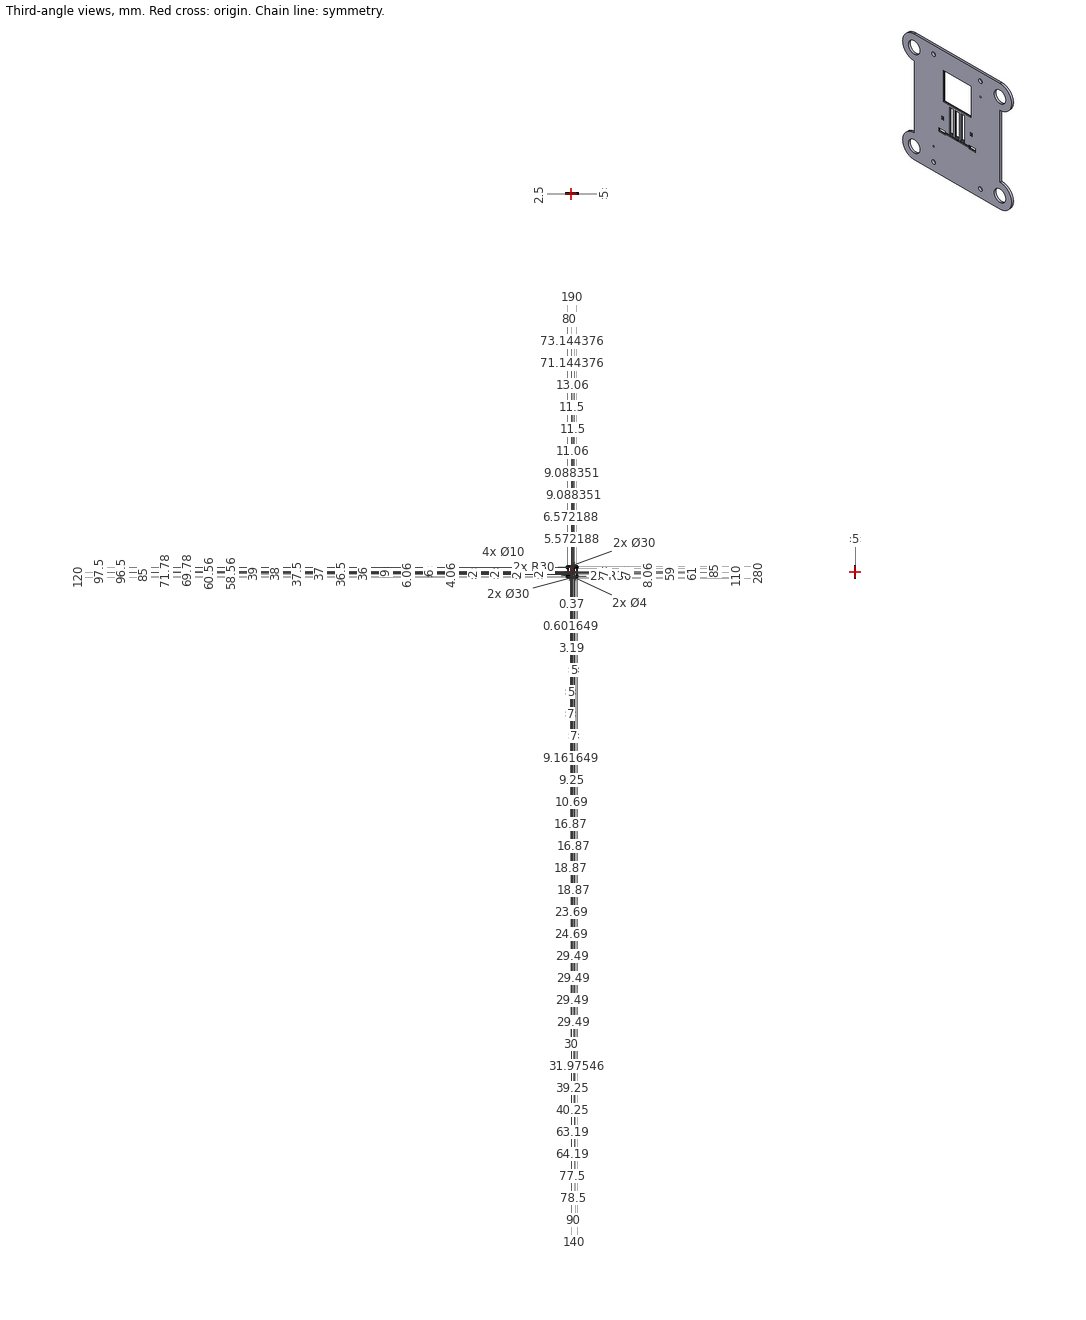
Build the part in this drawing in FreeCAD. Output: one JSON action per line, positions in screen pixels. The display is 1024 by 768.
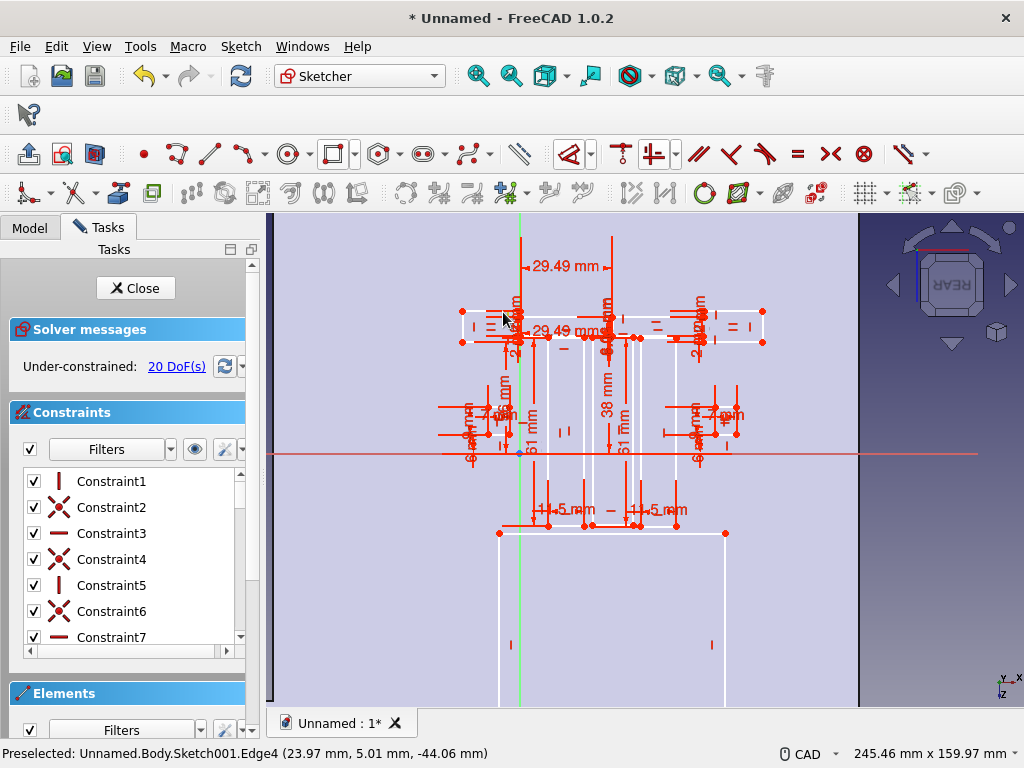
{"action": "left_click", "coordinate": [480, 311]}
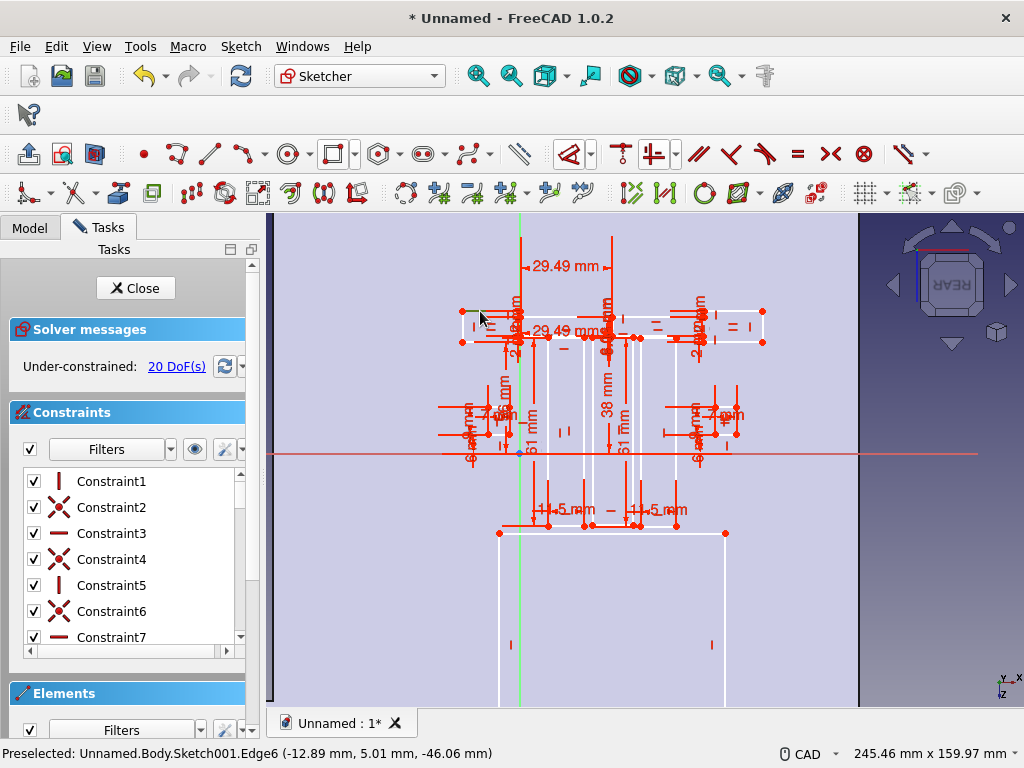
{"action": "key", "text": "l"}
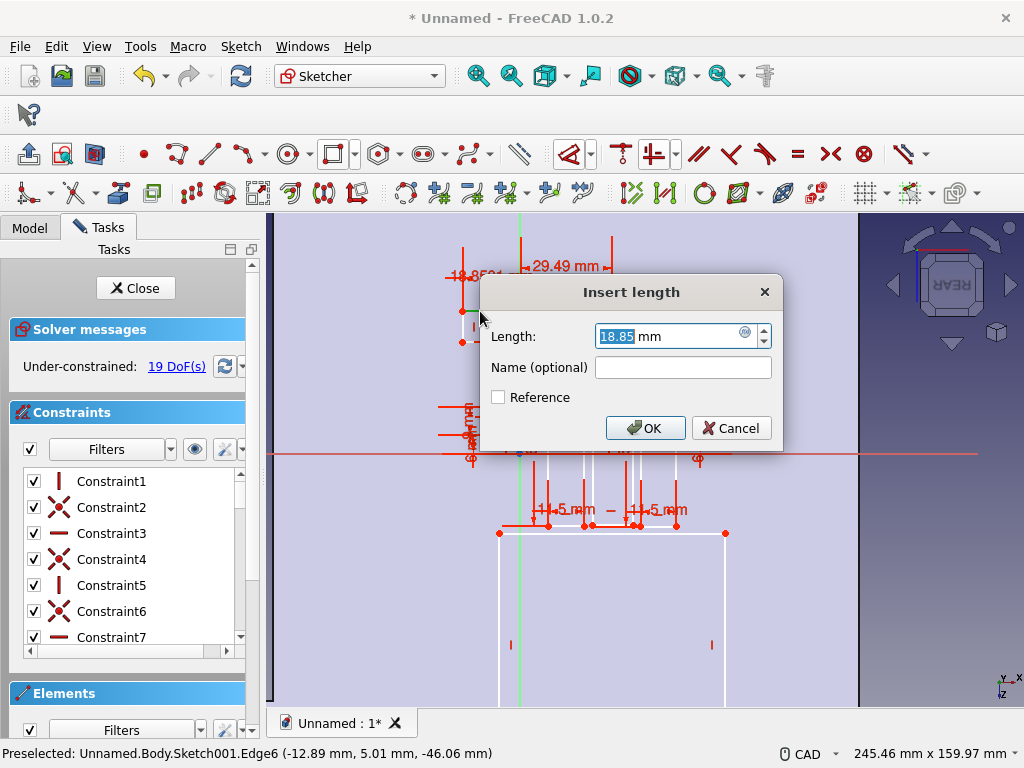
{"action": "type", "text": "18.87"}
{"action": "key", "text": "Return"}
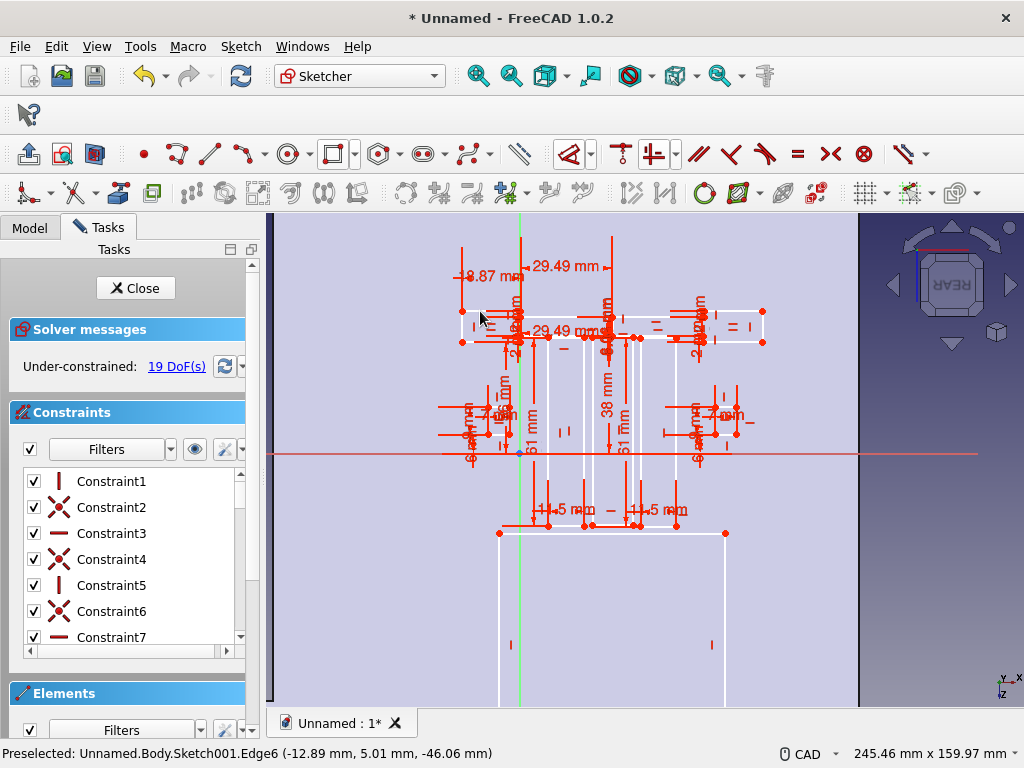
{"action": "left_click", "coordinate": [499, 600]}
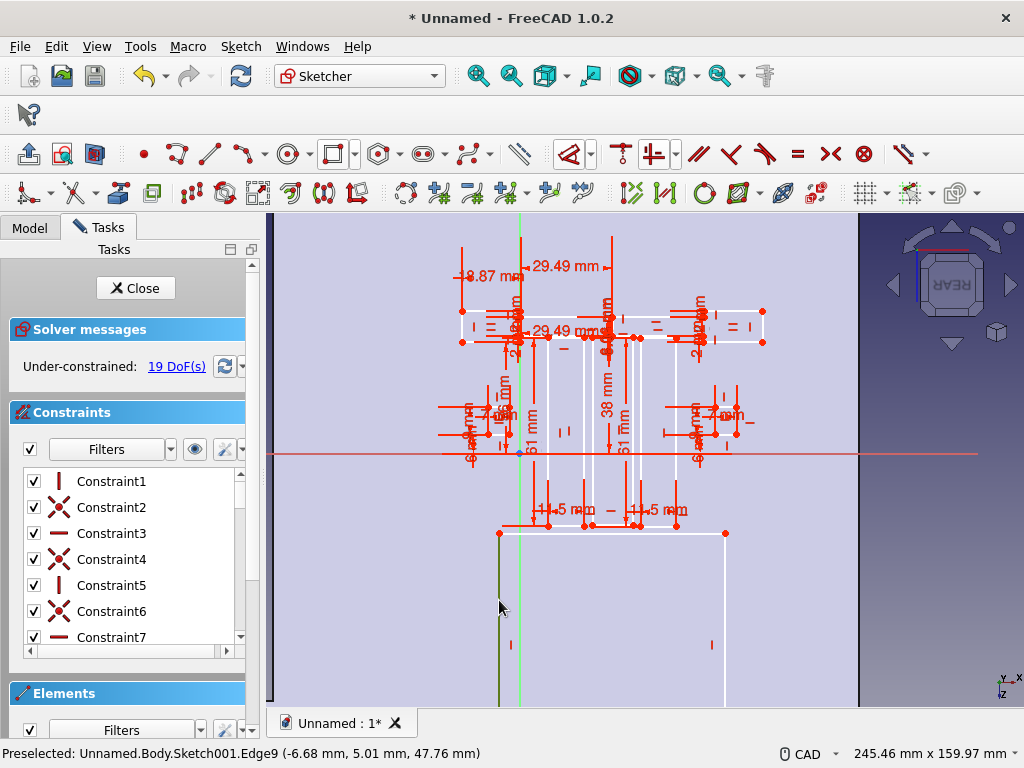
{"action": "key", "text": "i"}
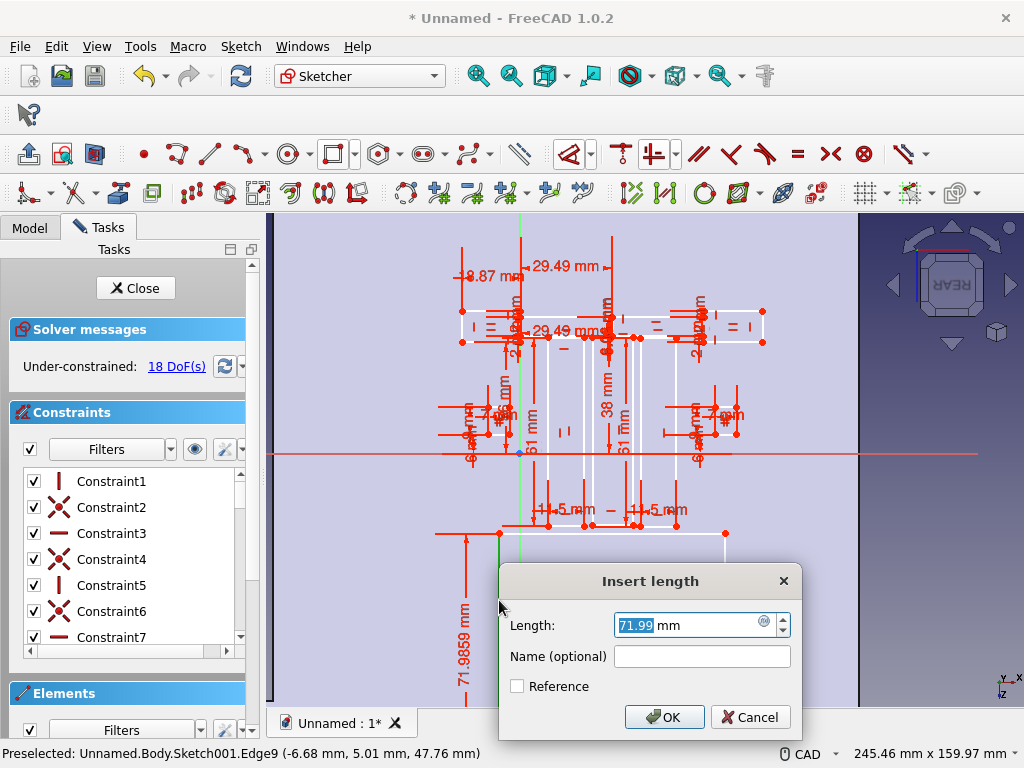
{"action": "type", "text": "71.78"}
{"action": "key", "text": "Return"}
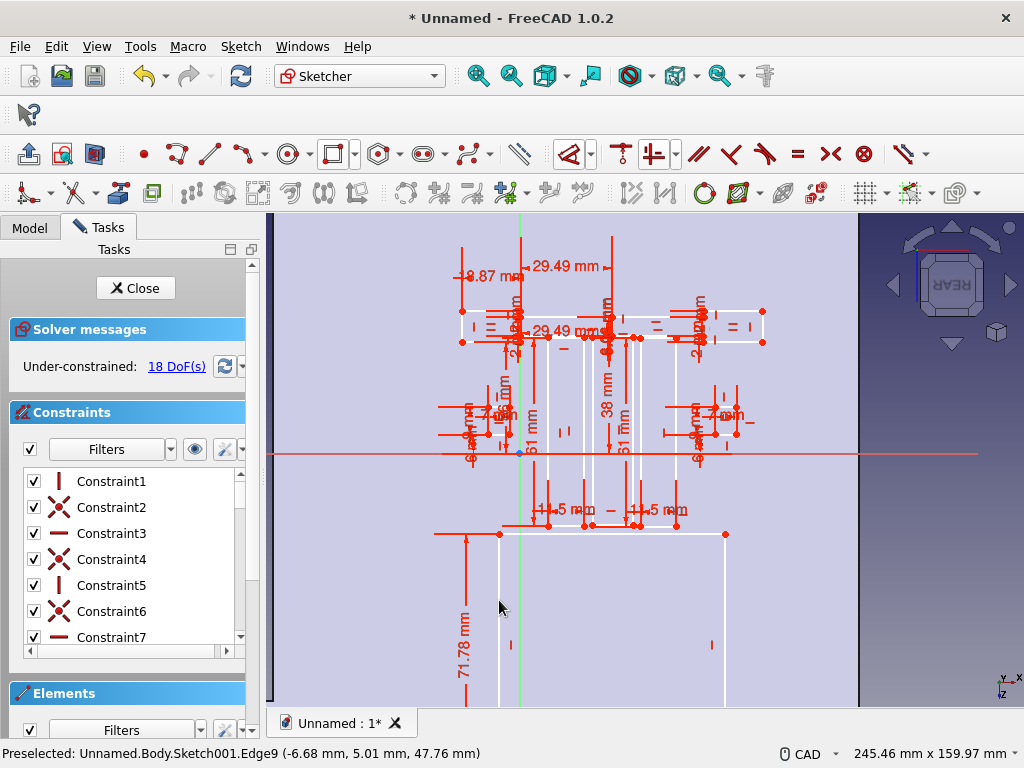
{"action": "scroll", "coordinate": [593, 394], "scroll_direction": "up", "scroll_amount": 3}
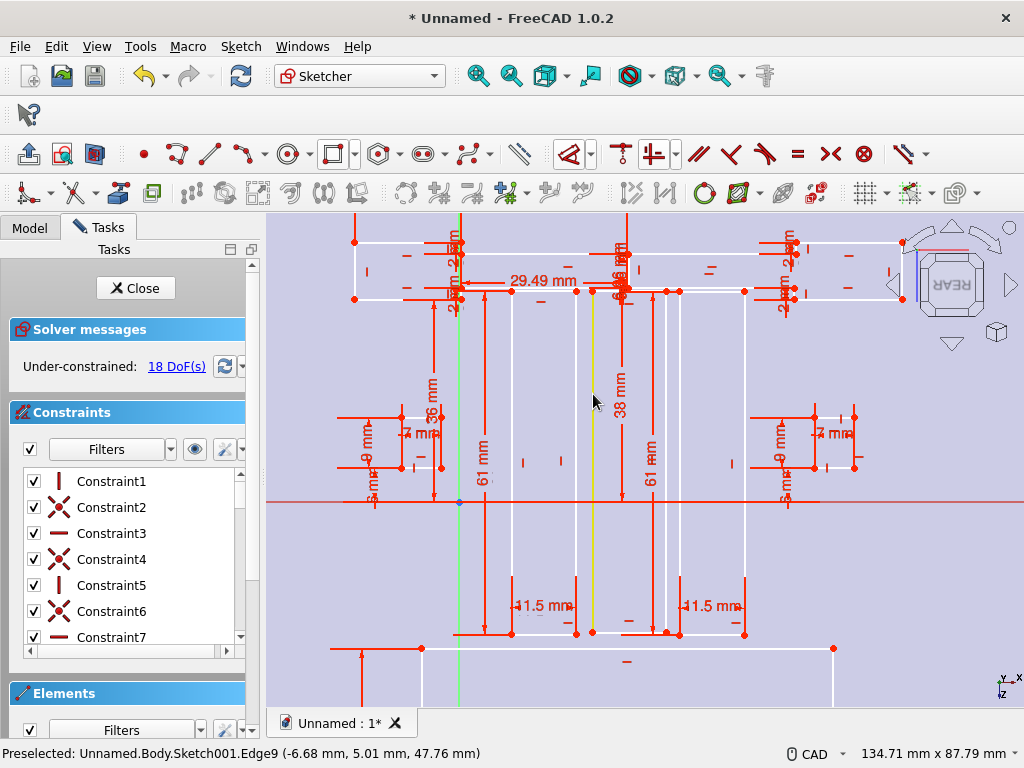
{"action": "left_click", "coordinate": [593, 394]}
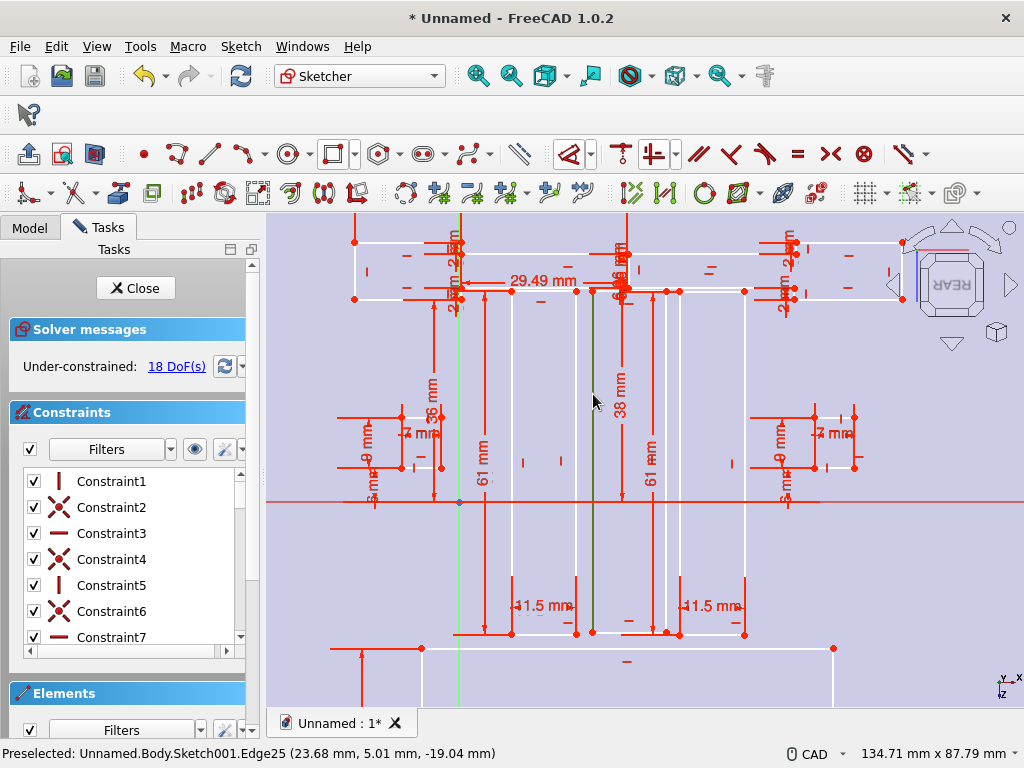
{"action": "key", "text": "i"}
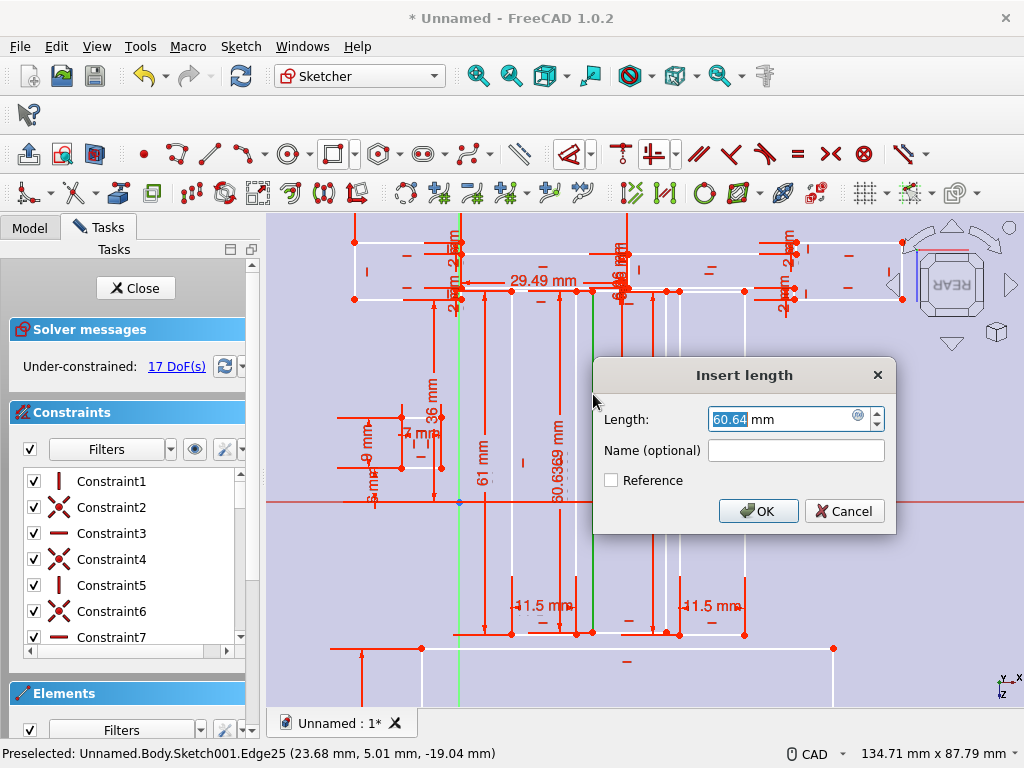
{"action": "type", "text": "60.56"}
{"action": "key", "text": "Return"}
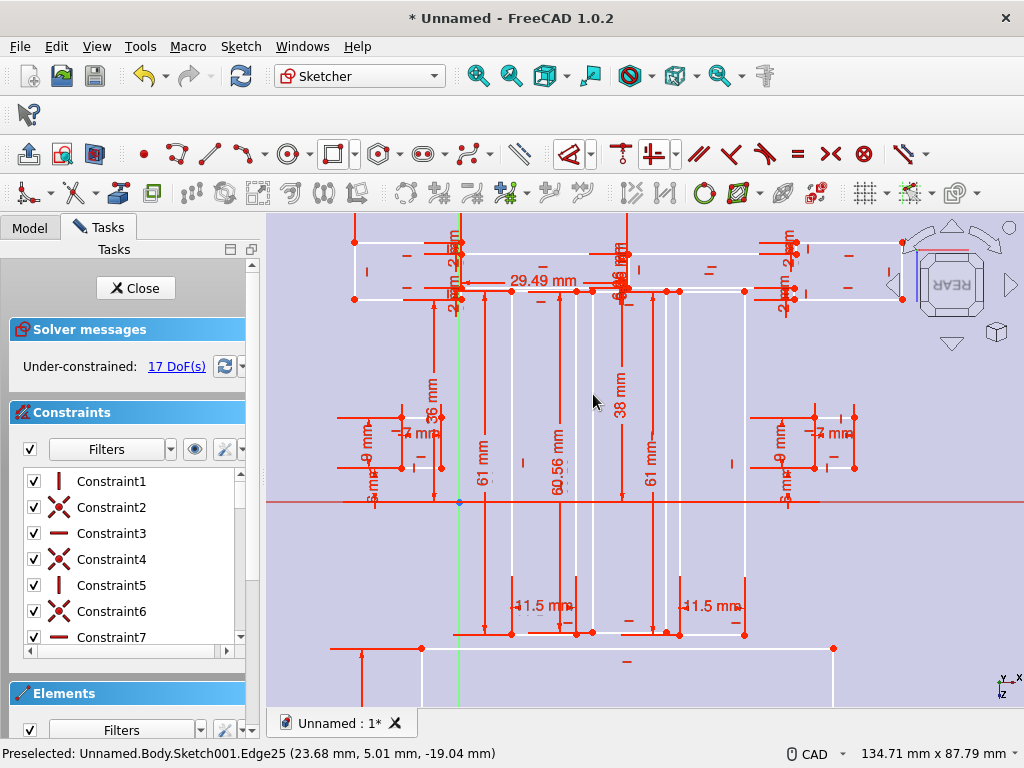
{"action": "left_click", "coordinate": [615, 633]}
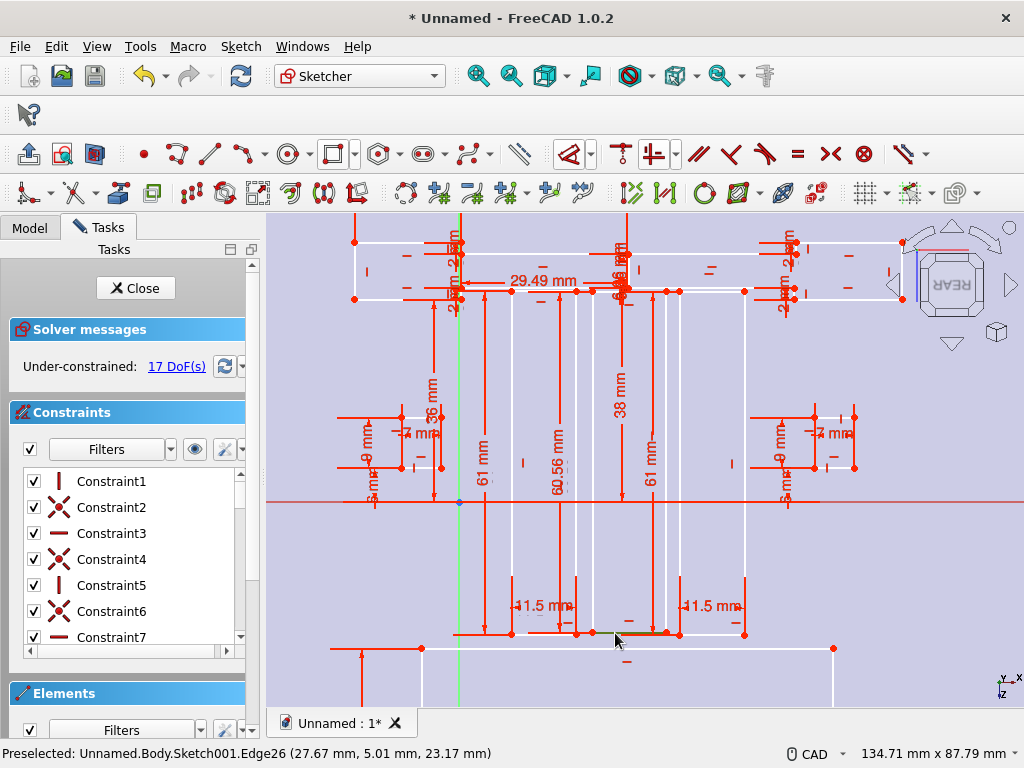
{"action": "key", "text": "l"}